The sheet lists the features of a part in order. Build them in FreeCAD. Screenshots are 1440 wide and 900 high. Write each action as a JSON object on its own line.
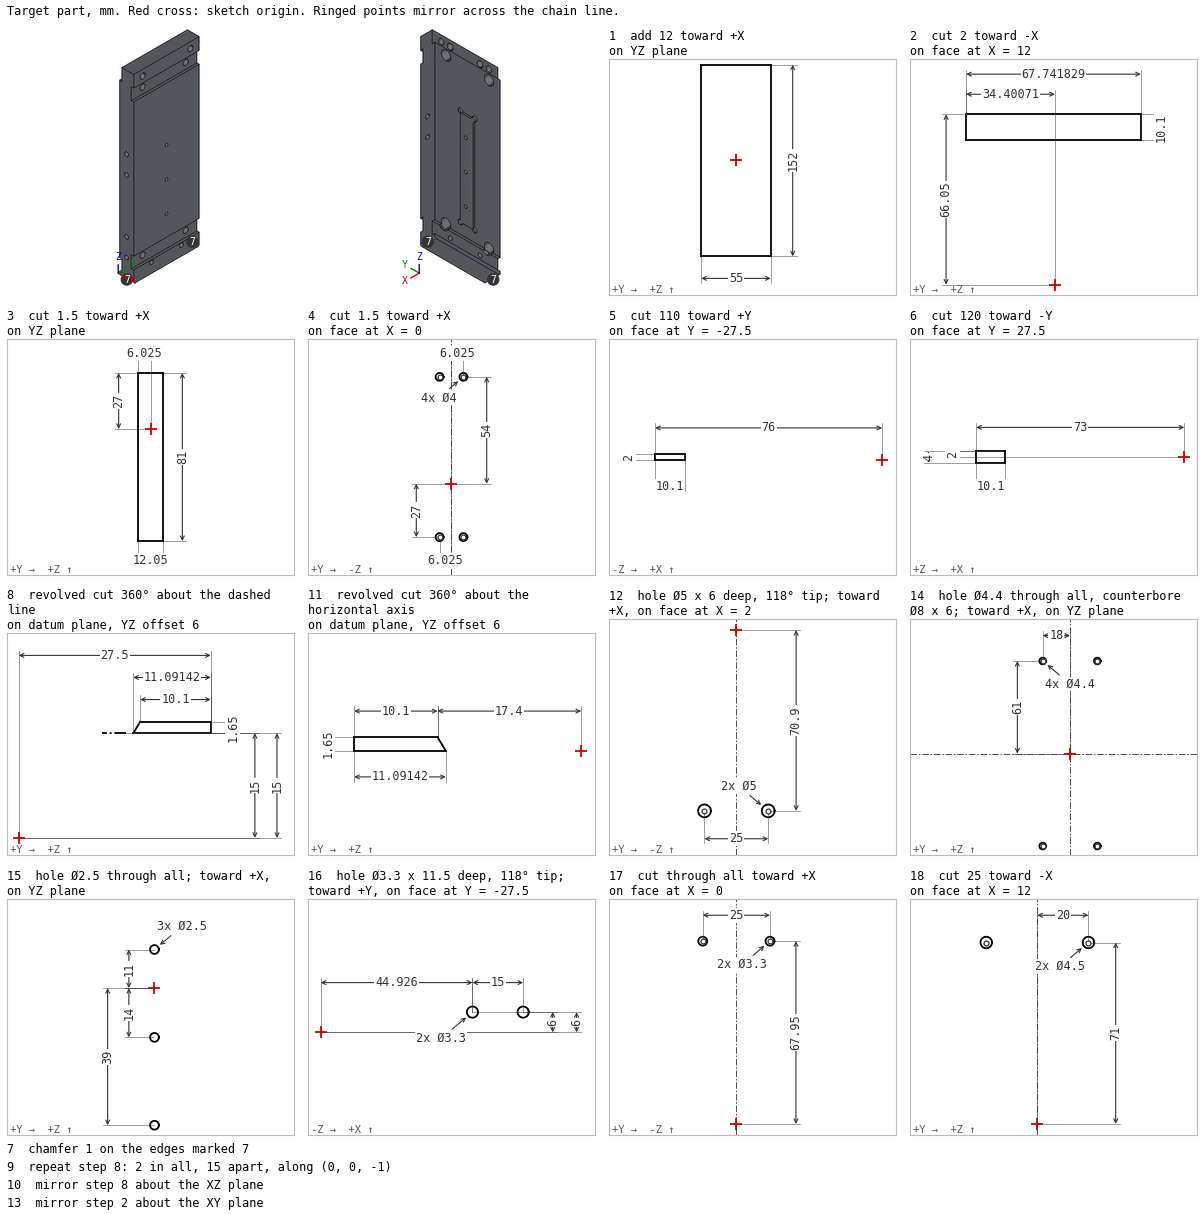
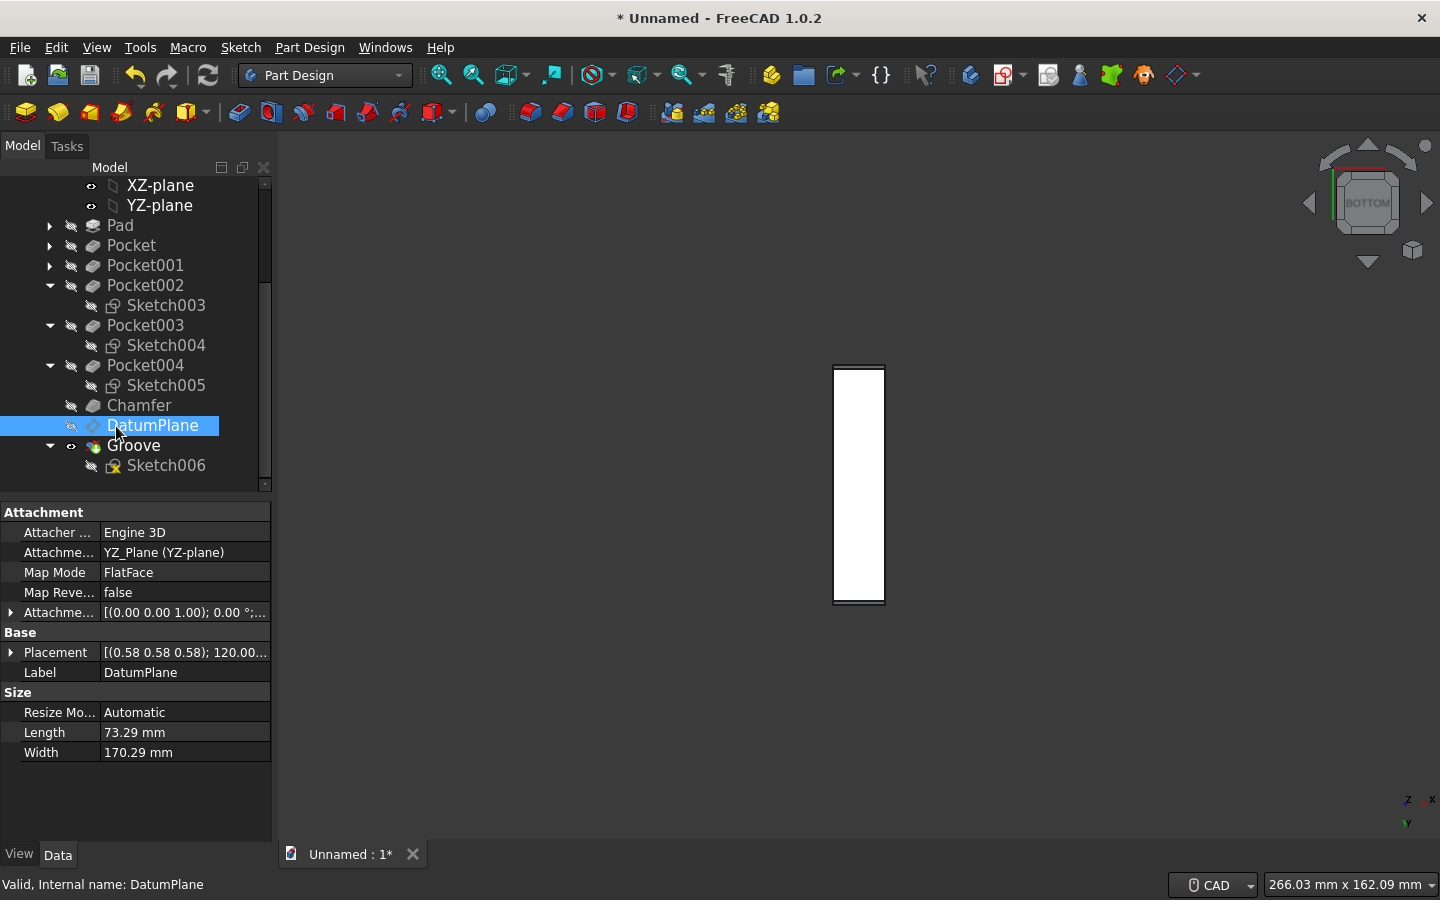
{"action": "left_click", "coordinate": [116, 446]}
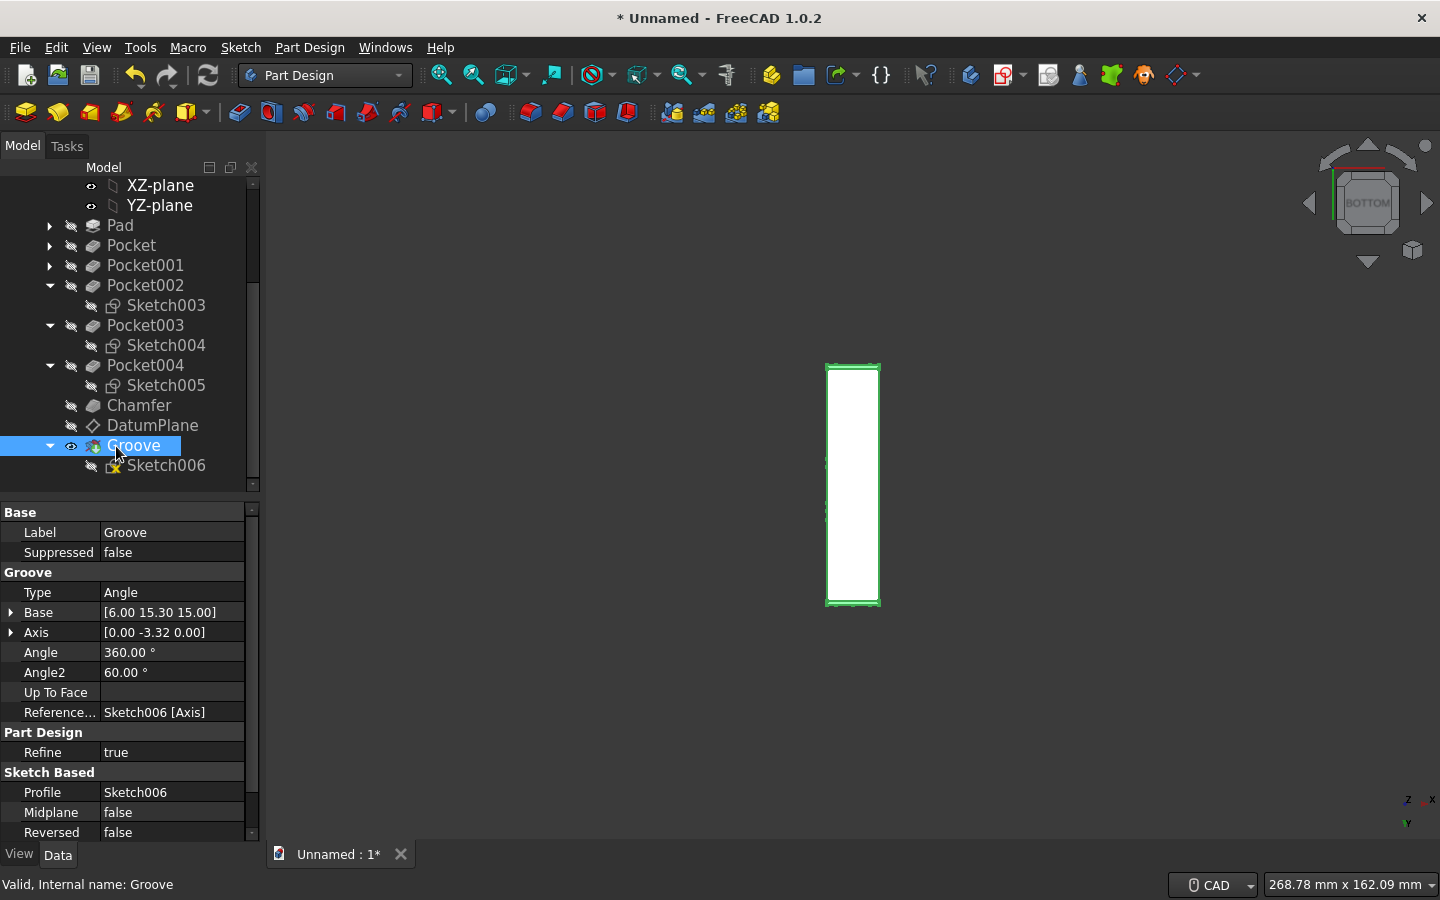
{"action": "left_click", "coordinate": [704, 112]}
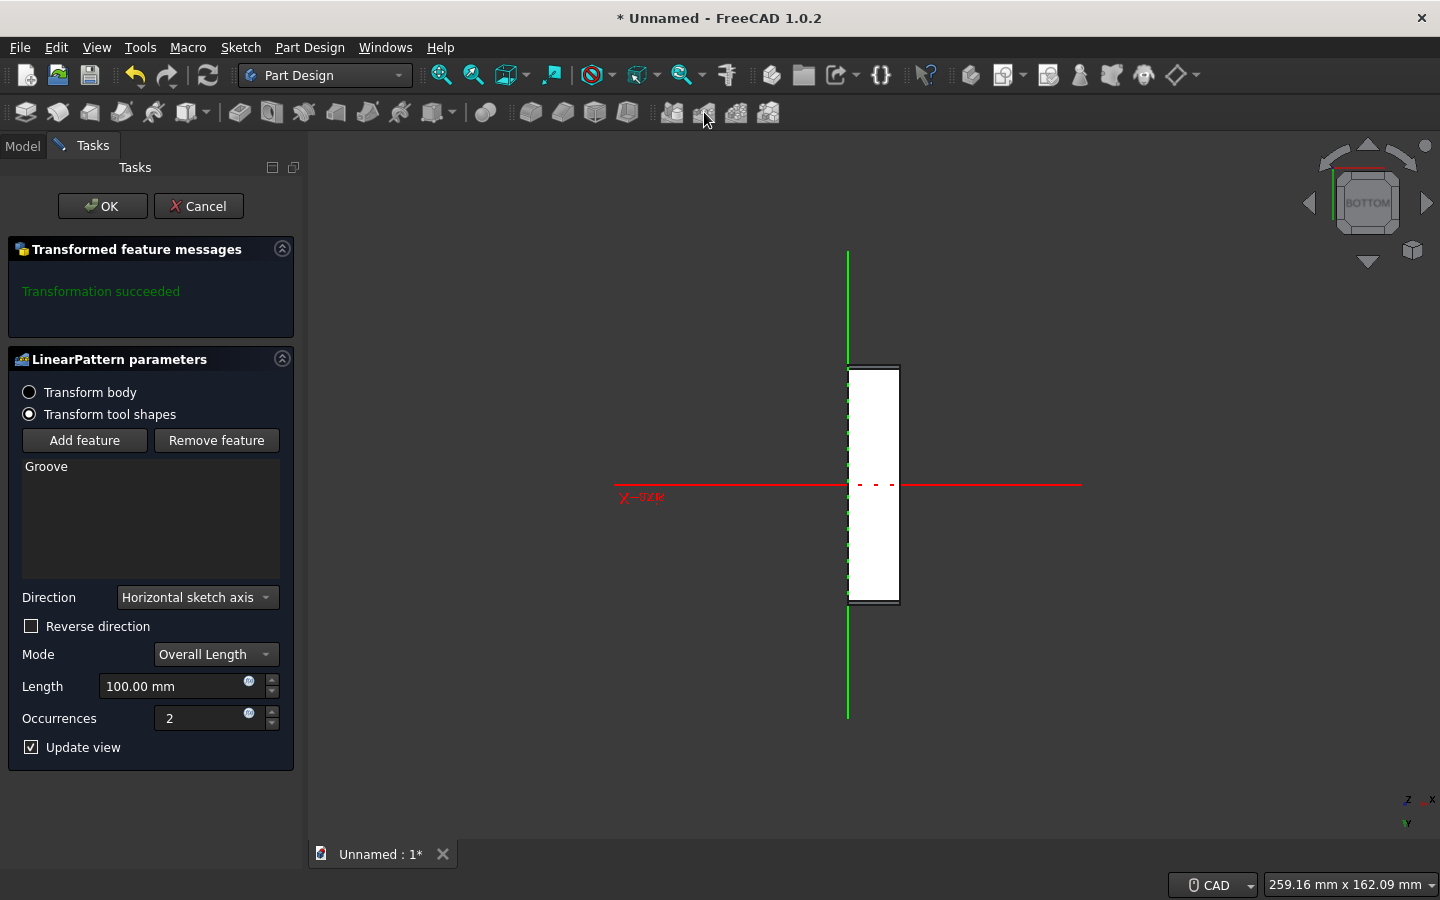
{"action": "left_click", "coordinate": [198, 598]}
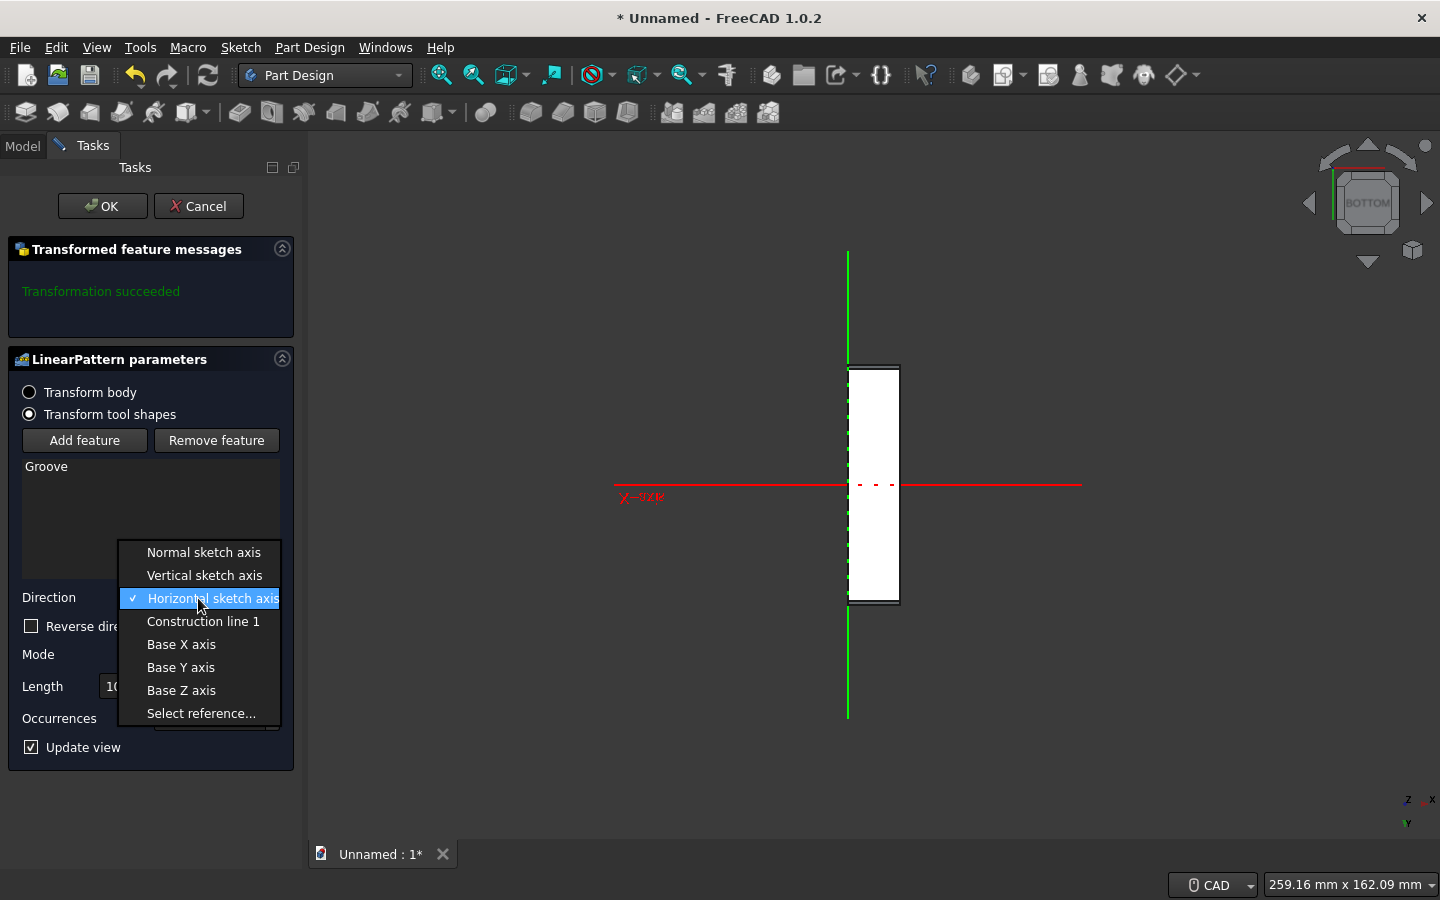
{"action": "left_click", "coordinate": [198, 690]}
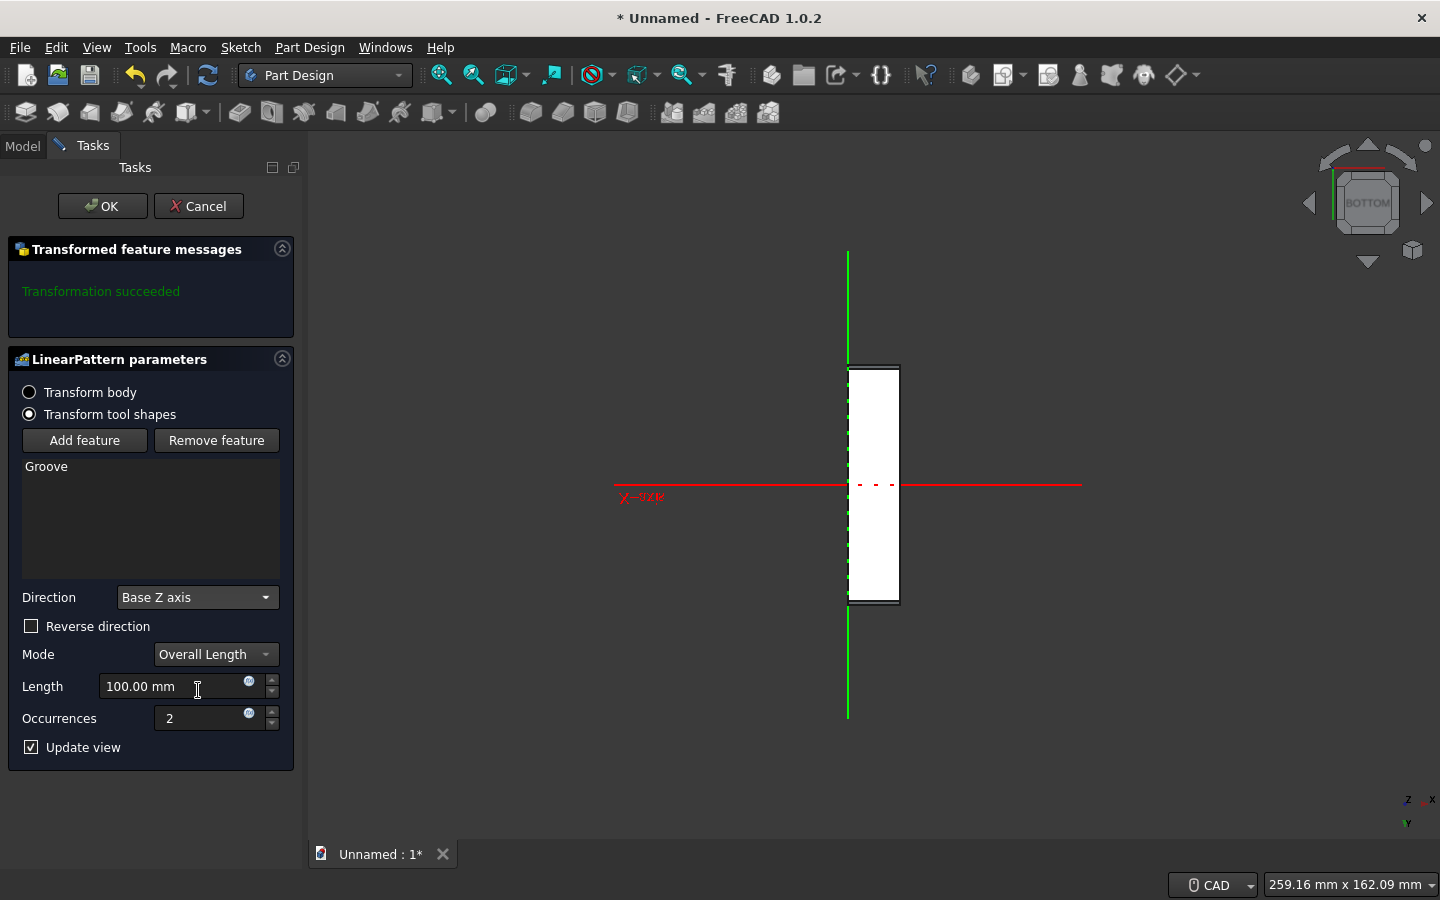
{"action": "left_click", "coordinate": [217, 654]}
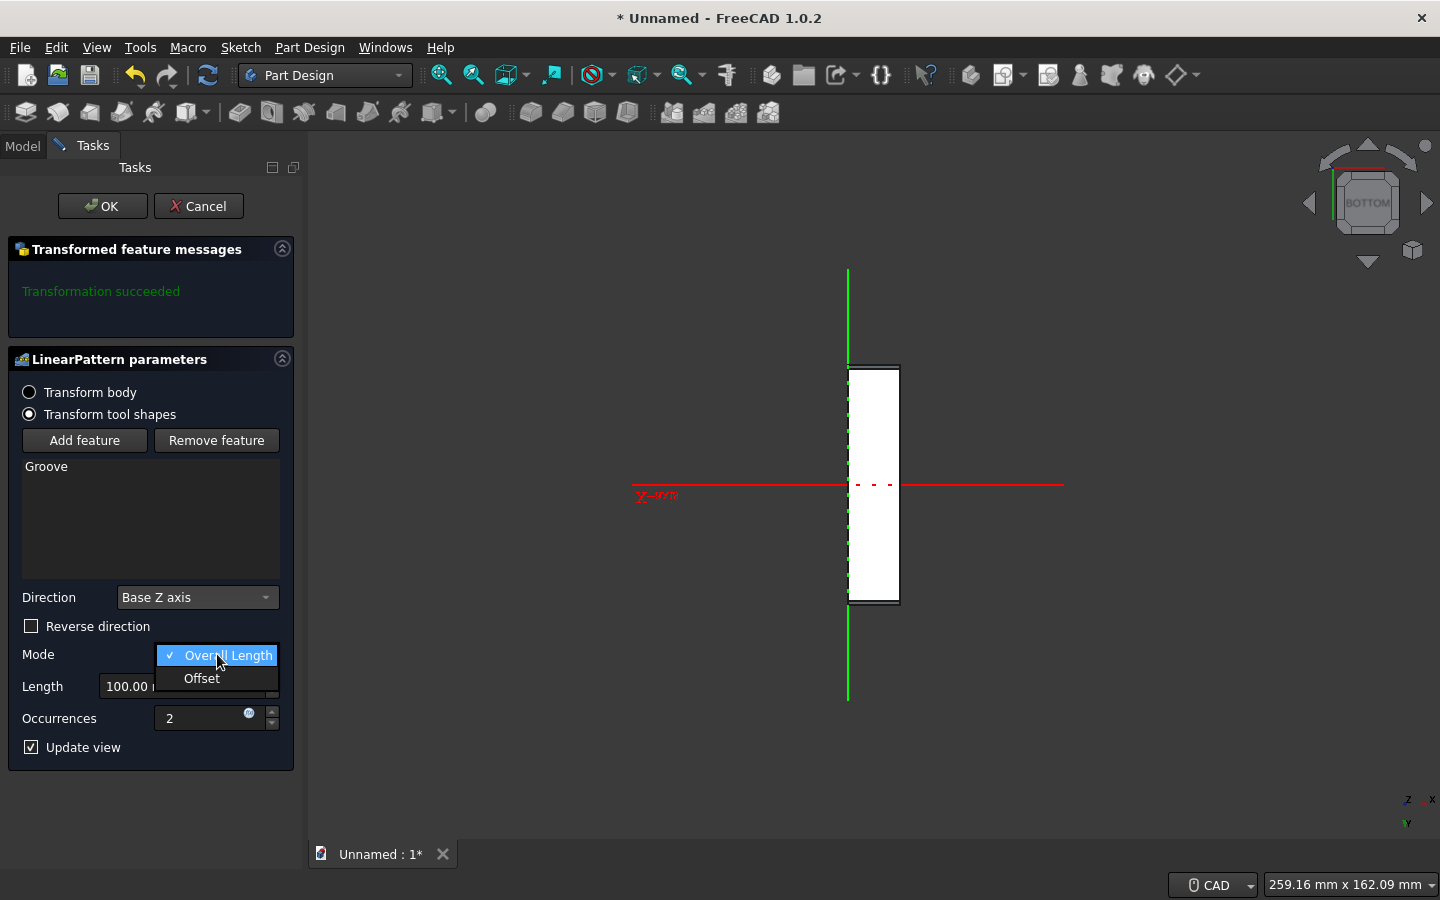
{"action": "left_click", "coordinate": [216, 678]}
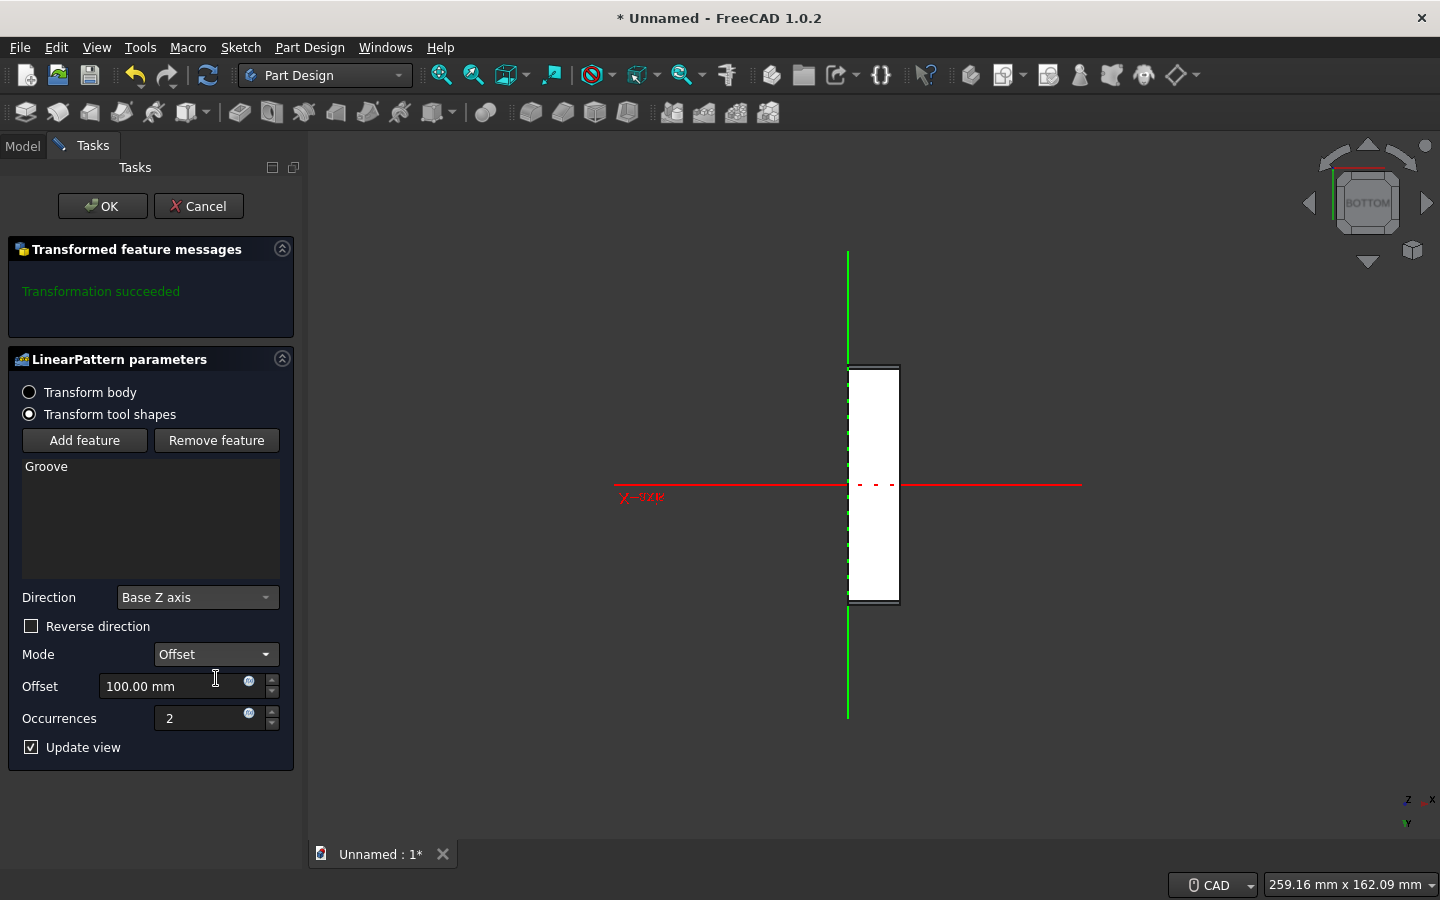
{"action": "triple_click", "coordinate": [182, 686]}